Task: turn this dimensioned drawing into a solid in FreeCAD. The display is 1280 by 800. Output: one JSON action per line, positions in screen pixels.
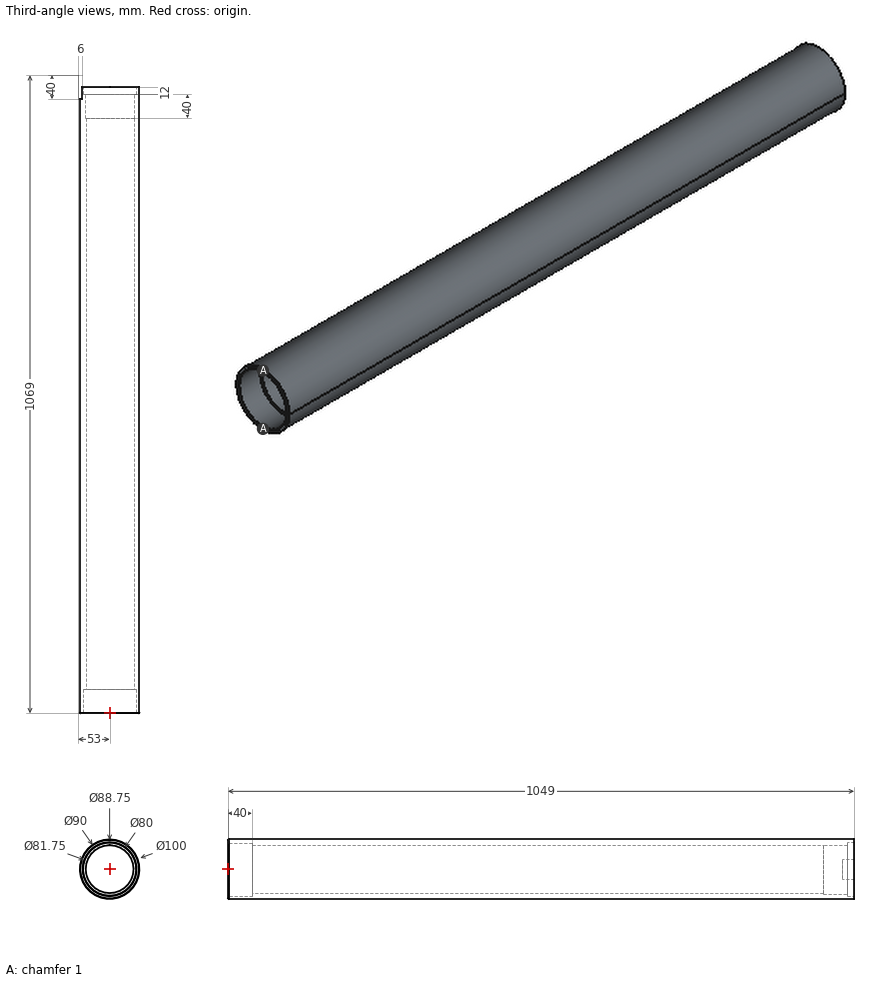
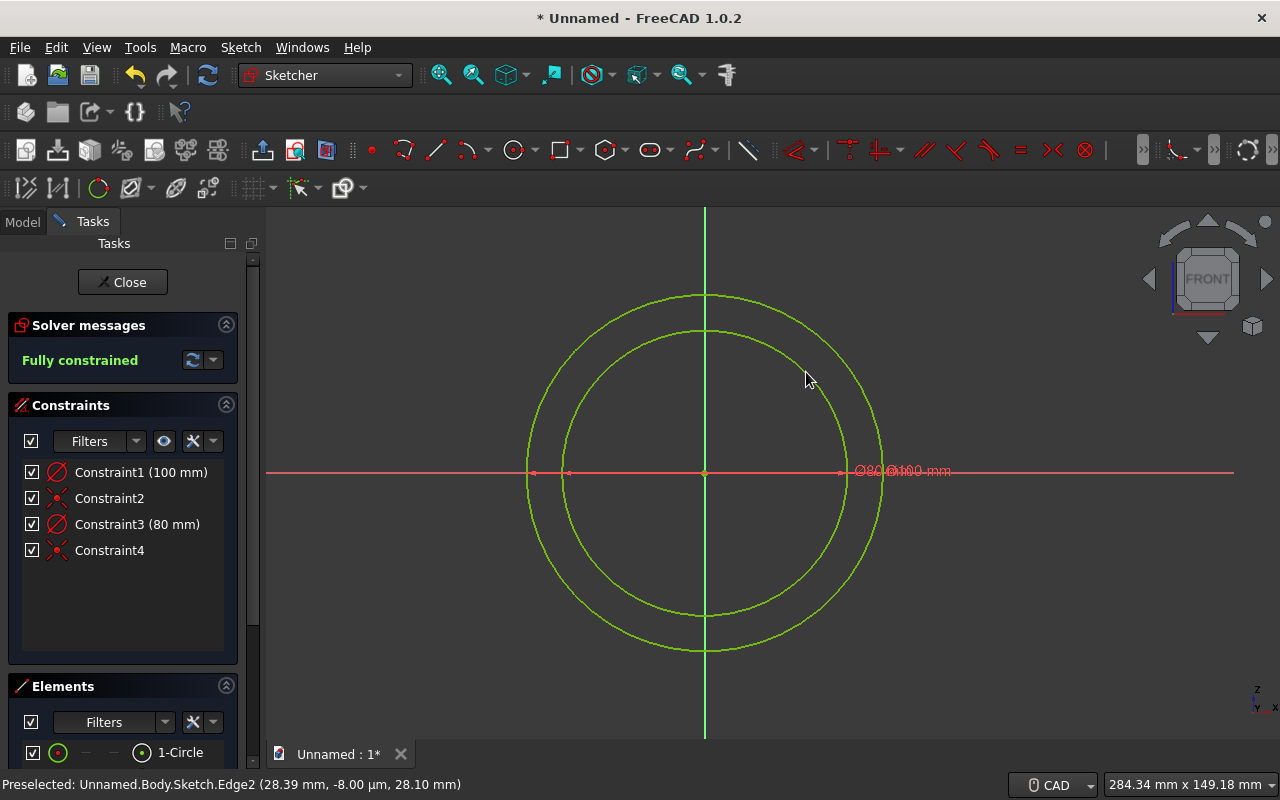
{"action": "left_click", "coordinate": [123, 282]}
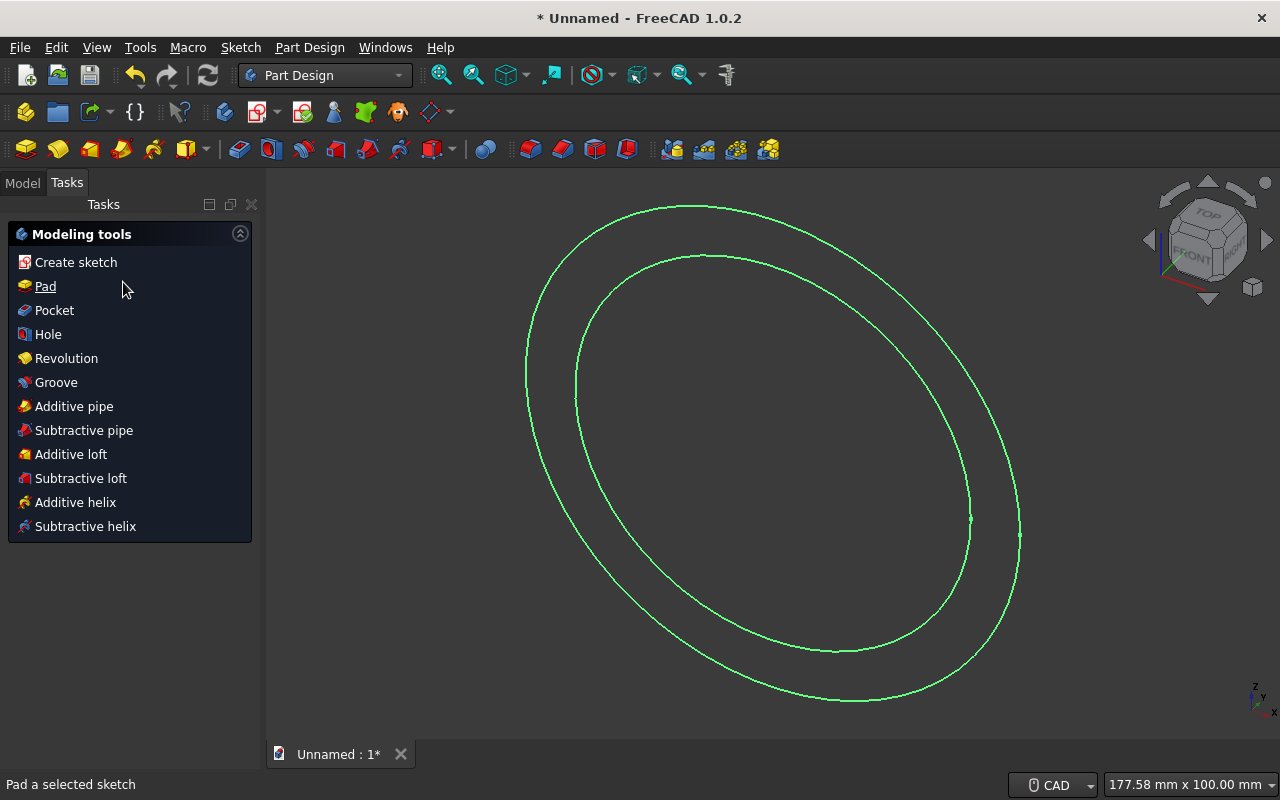
{"action": "left_click", "coordinate": [26, 150]}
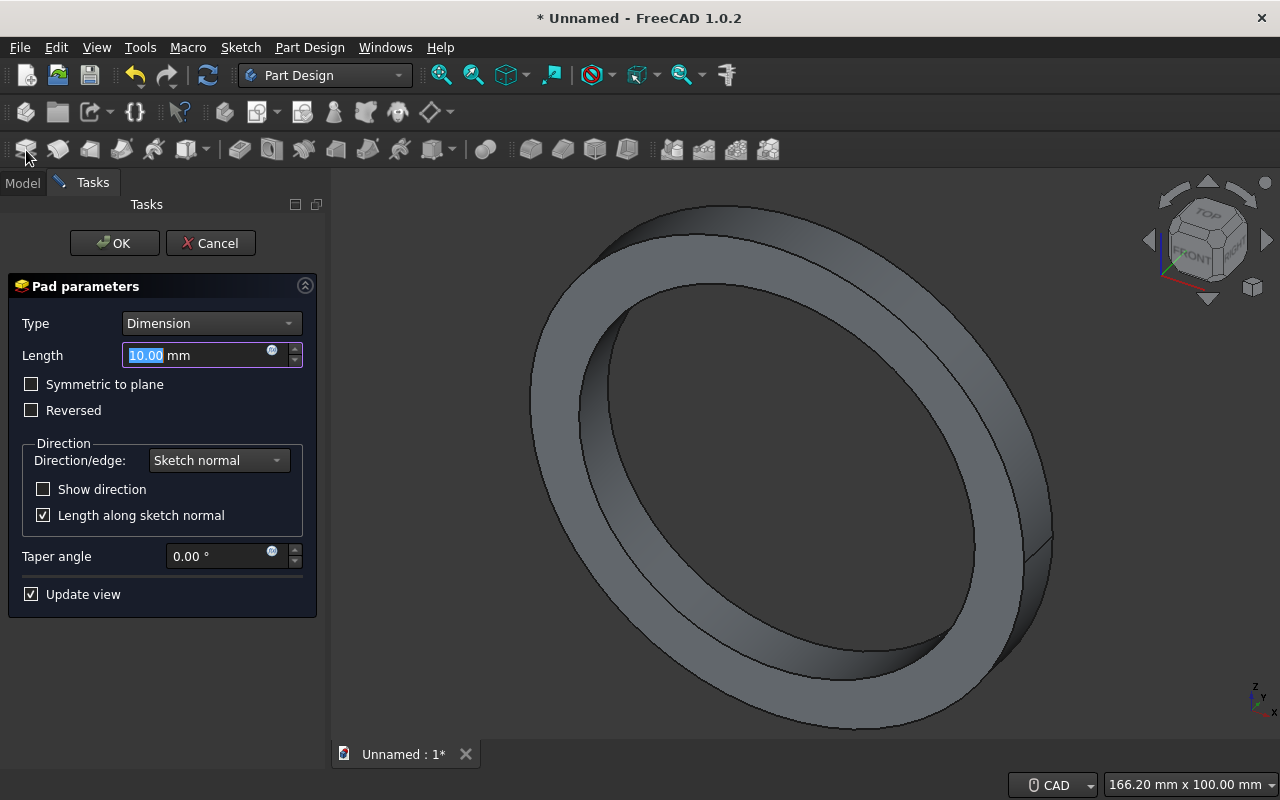
{"action": "type", "text": "1049"}
{"action": "key", "text": "Tab"}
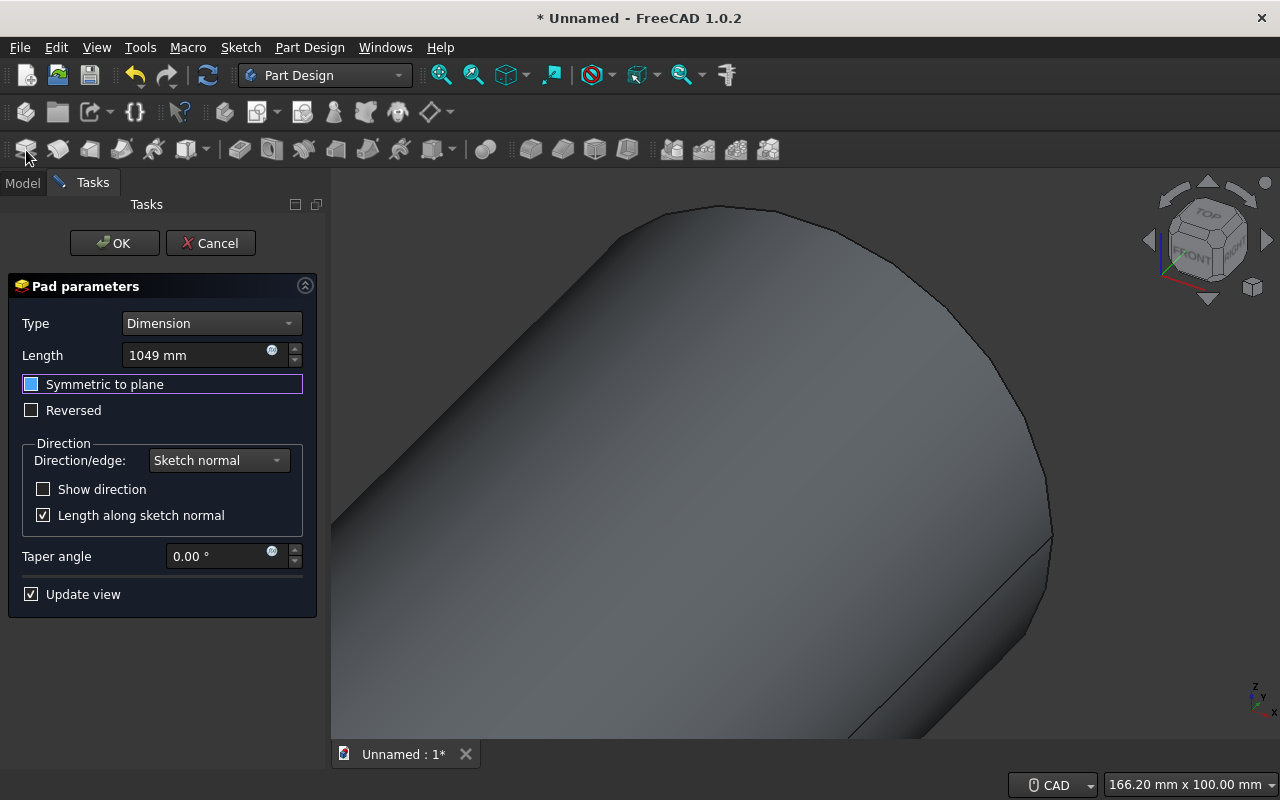
{"action": "left_click", "coordinate": [30, 410]}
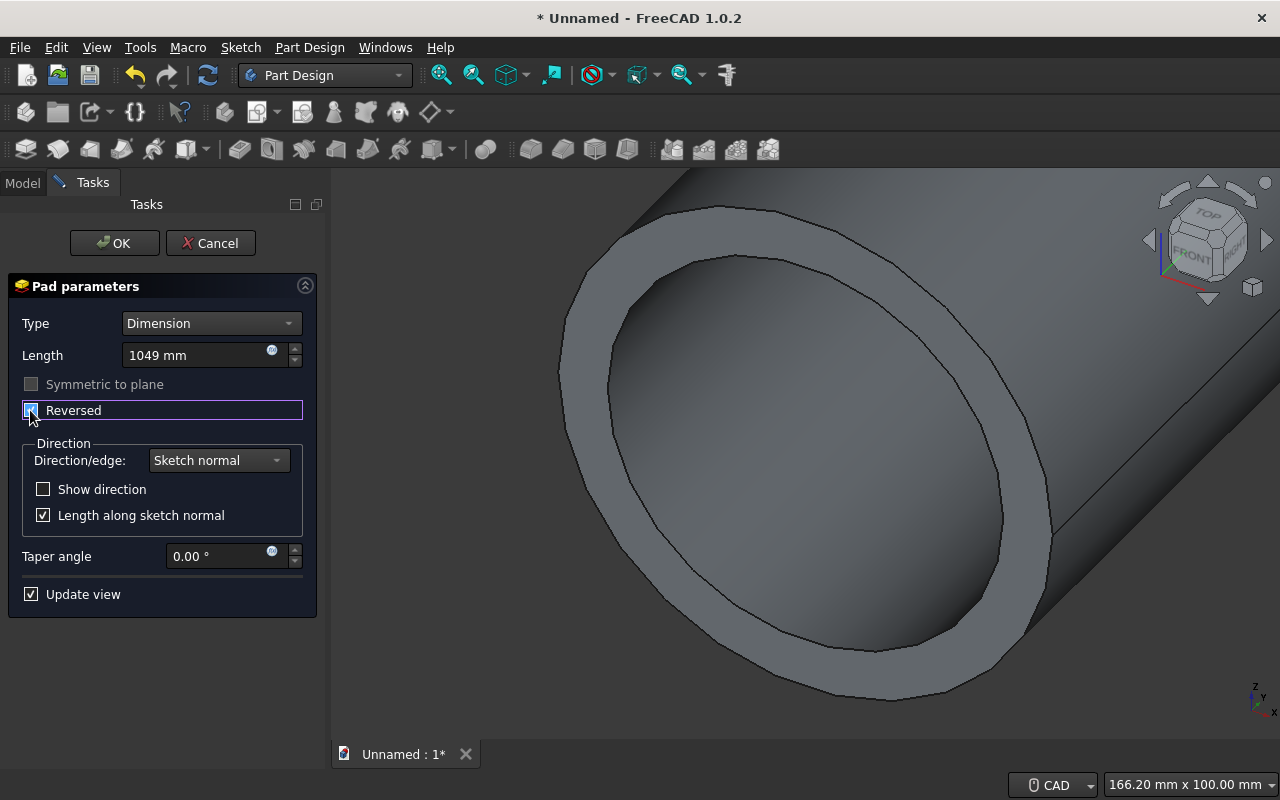
{"action": "left_click", "coordinate": [115, 243]}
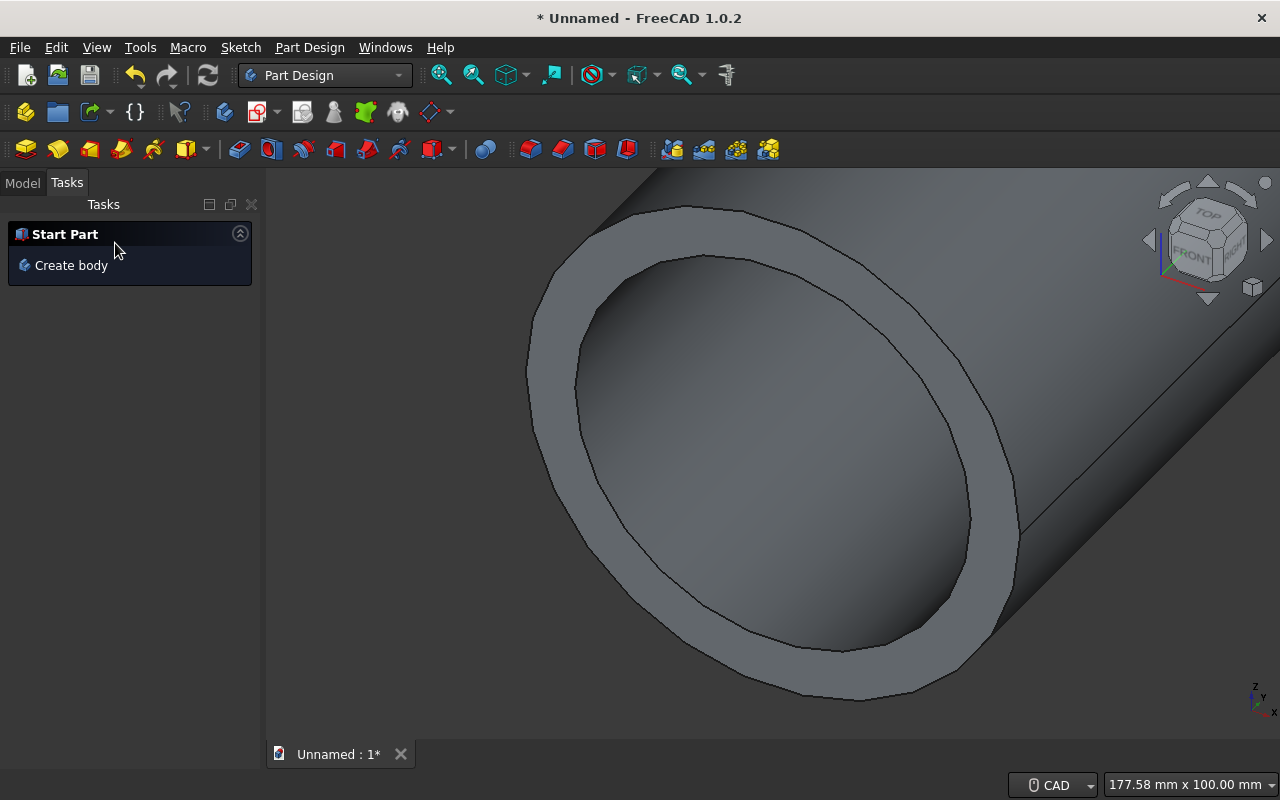
{"action": "left_click", "coordinate": [442, 76]}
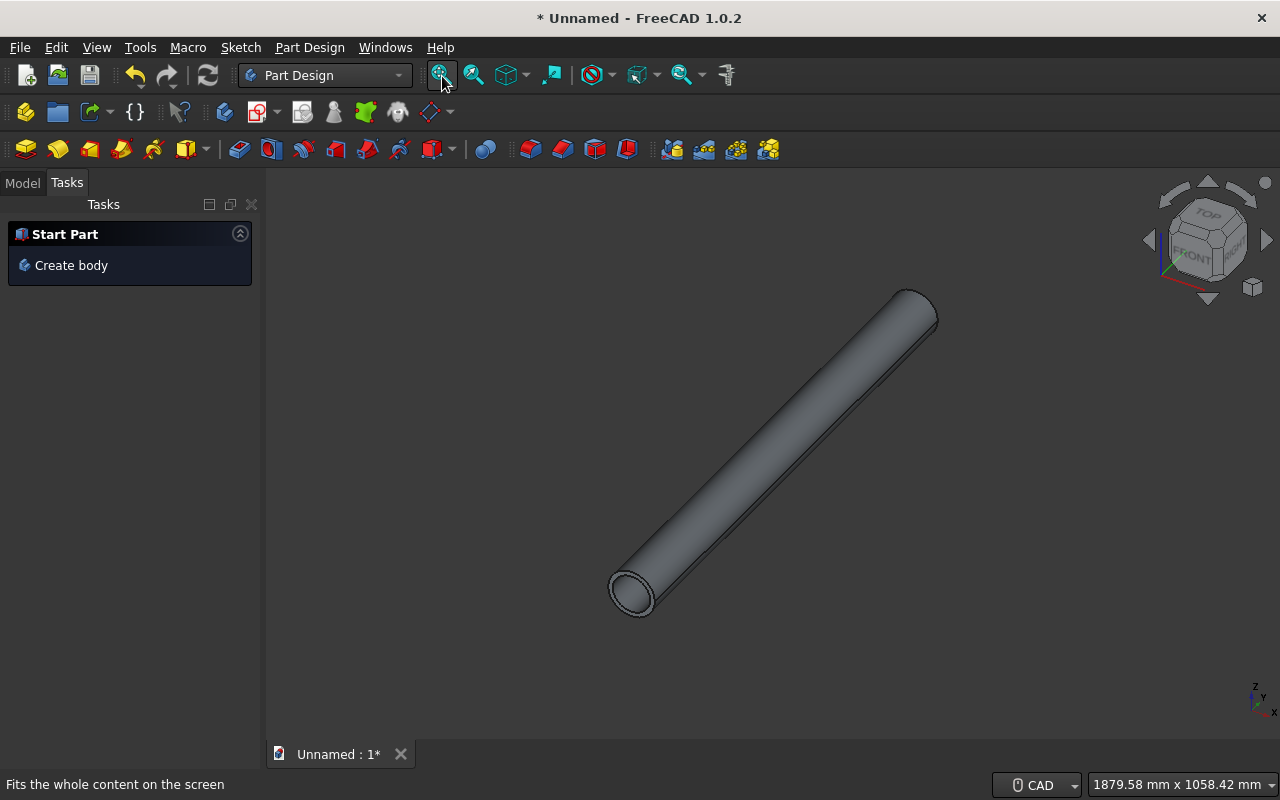
{"action": "key", "text": "4"}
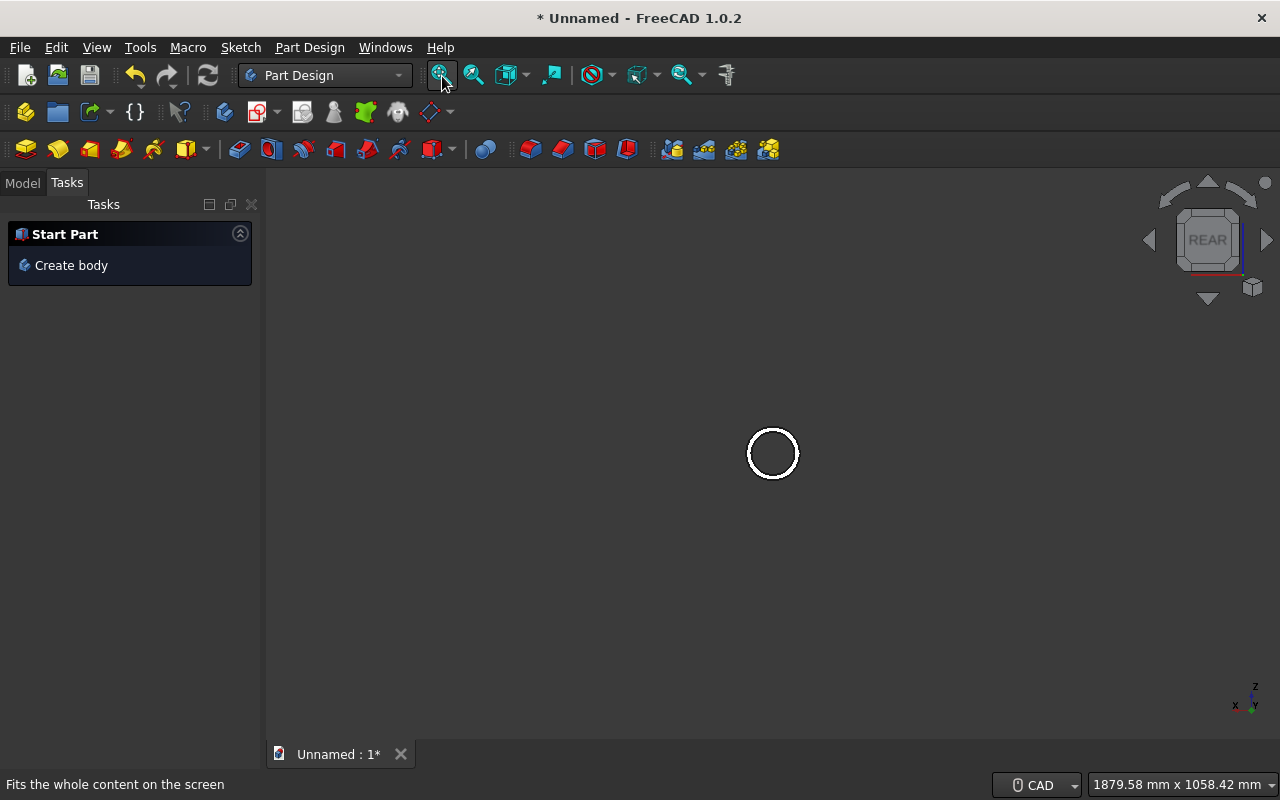
{"action": "left_click", "coordinate": [442, 76]}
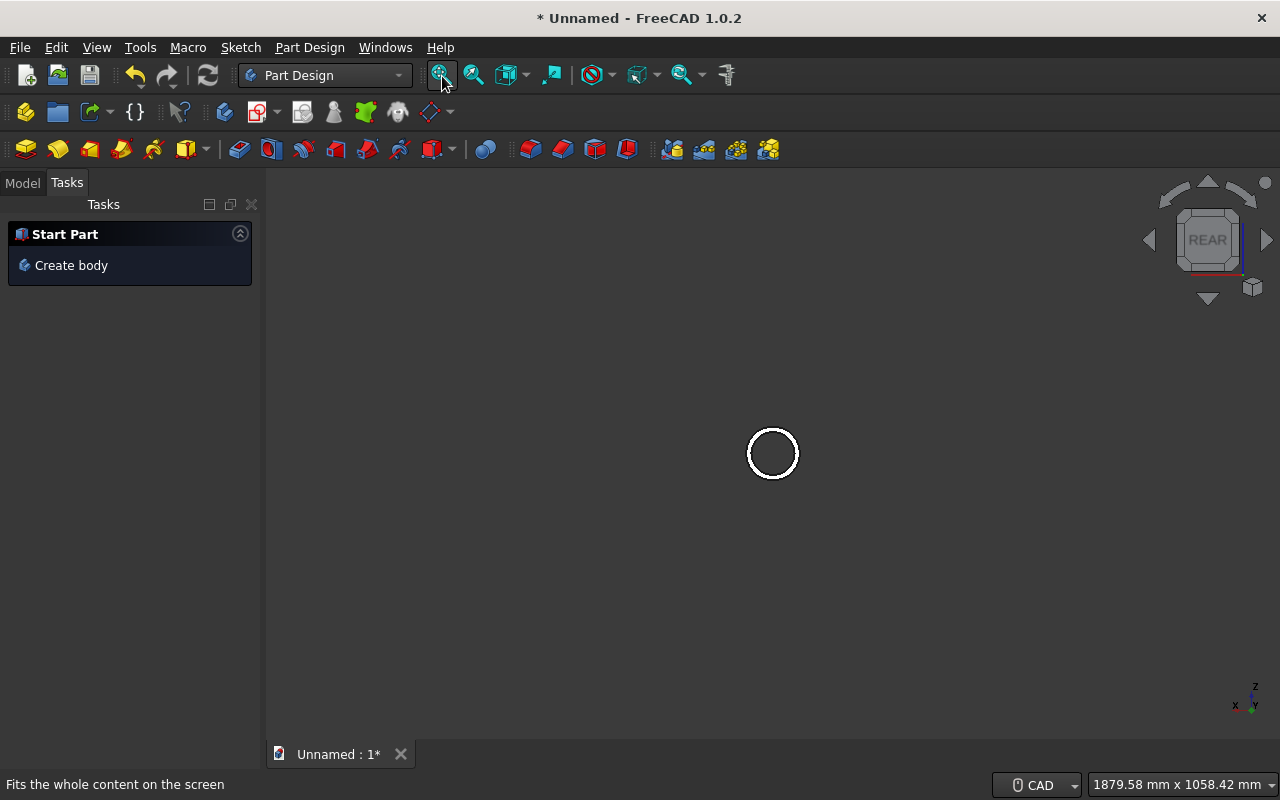
{"action": "scroll", "coordinate": [796, 460], "scroll_direction": "up", "scroll_amount": 8}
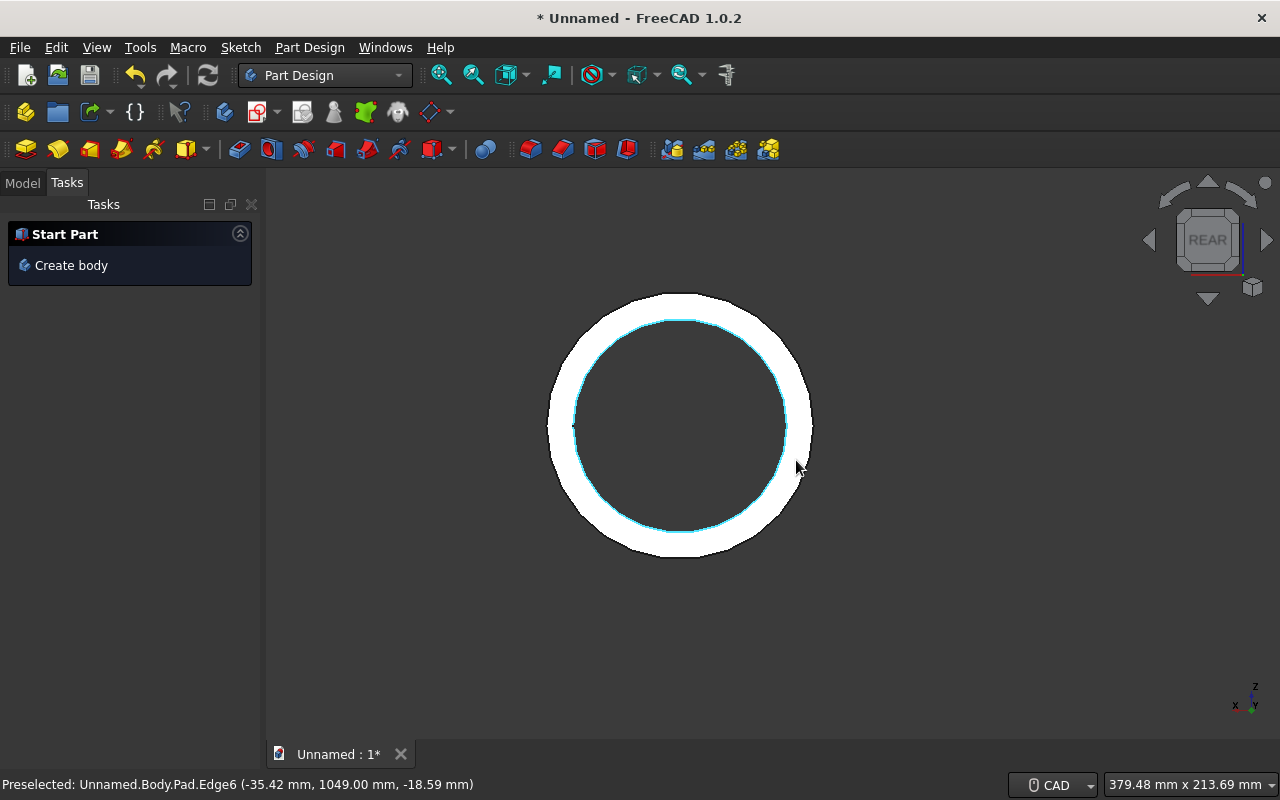
{"action": "left_click", "coordinate": [795, 463]}